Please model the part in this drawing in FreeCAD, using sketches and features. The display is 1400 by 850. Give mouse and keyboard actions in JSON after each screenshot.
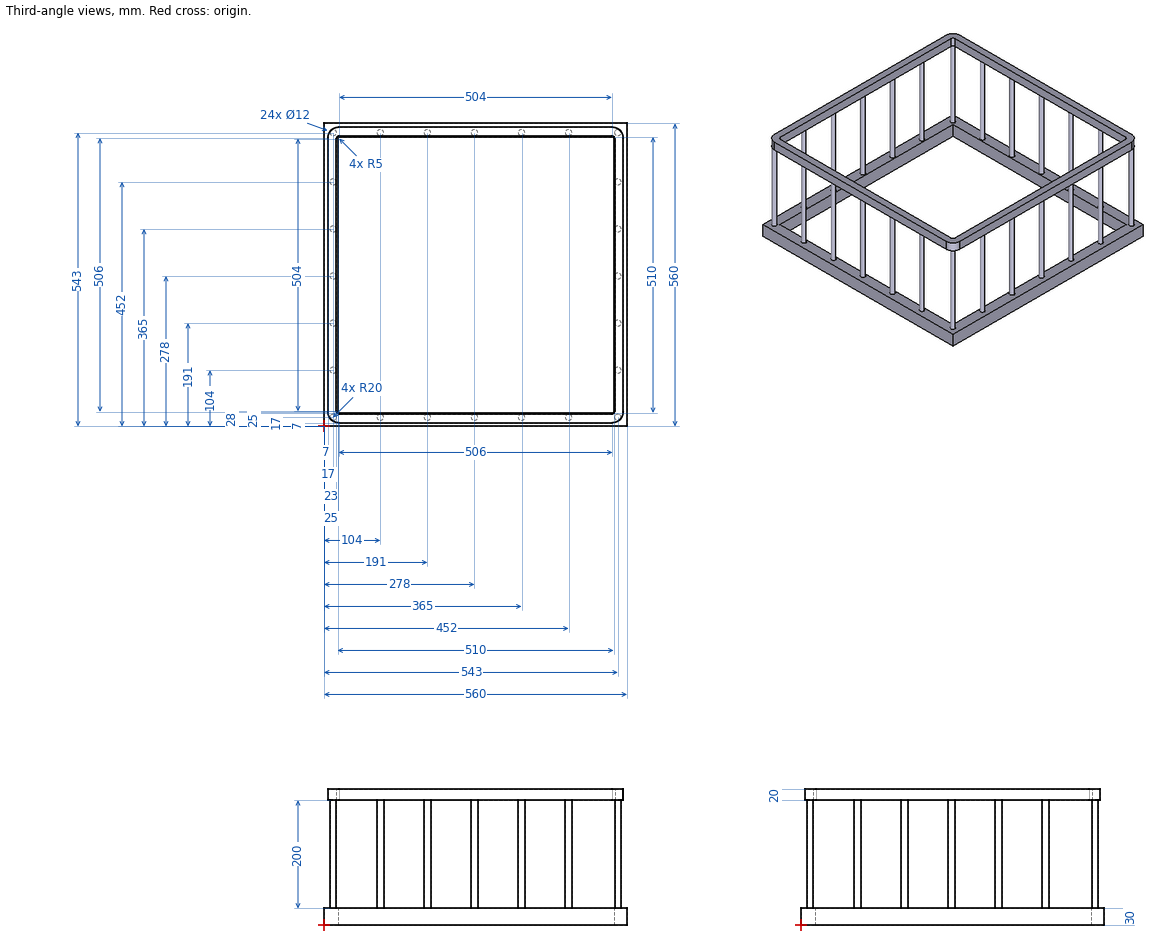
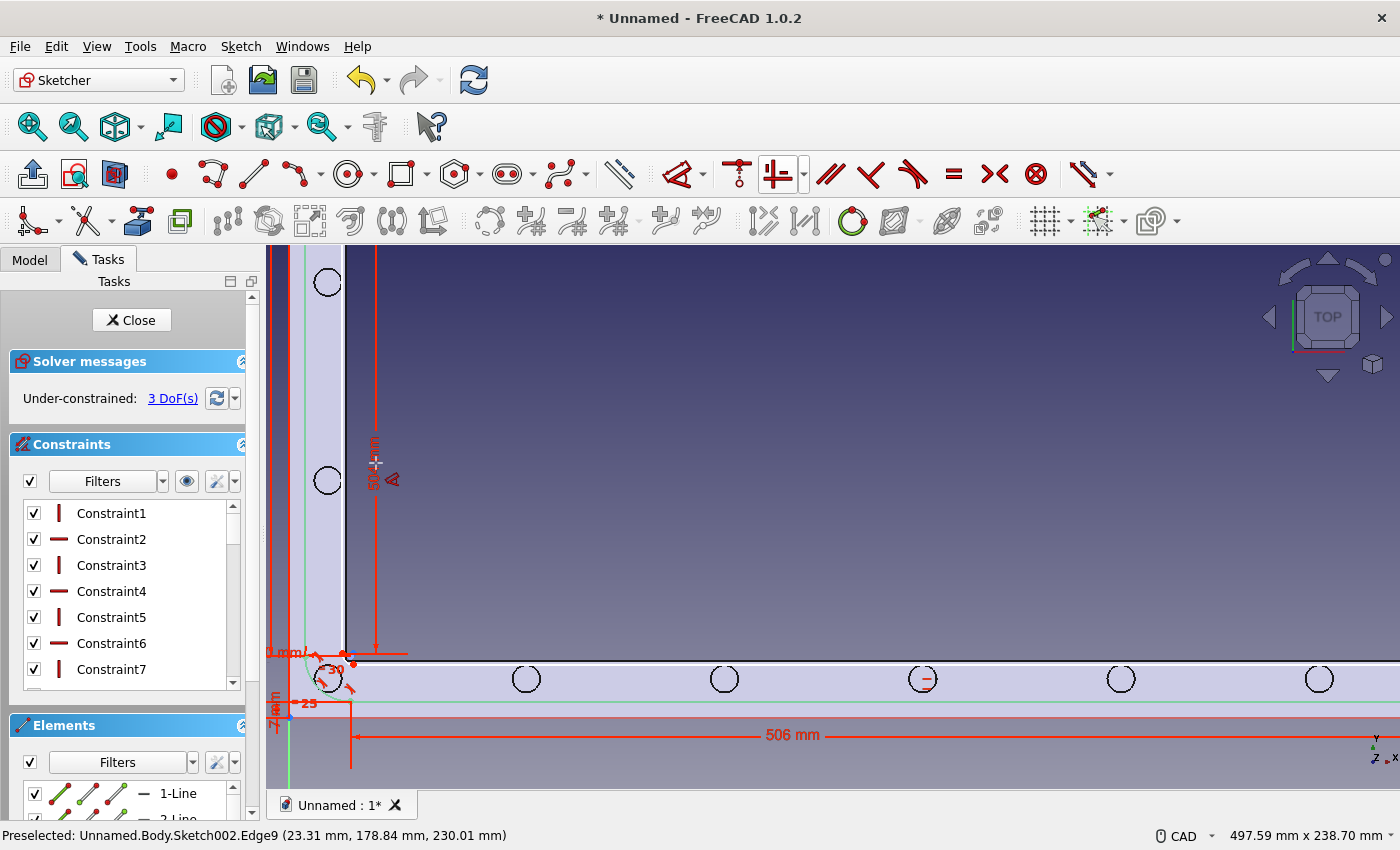
{"action": "scroll", "coordinate": [698, 702], "scroll_direction": "down", "scroll_amount": 6}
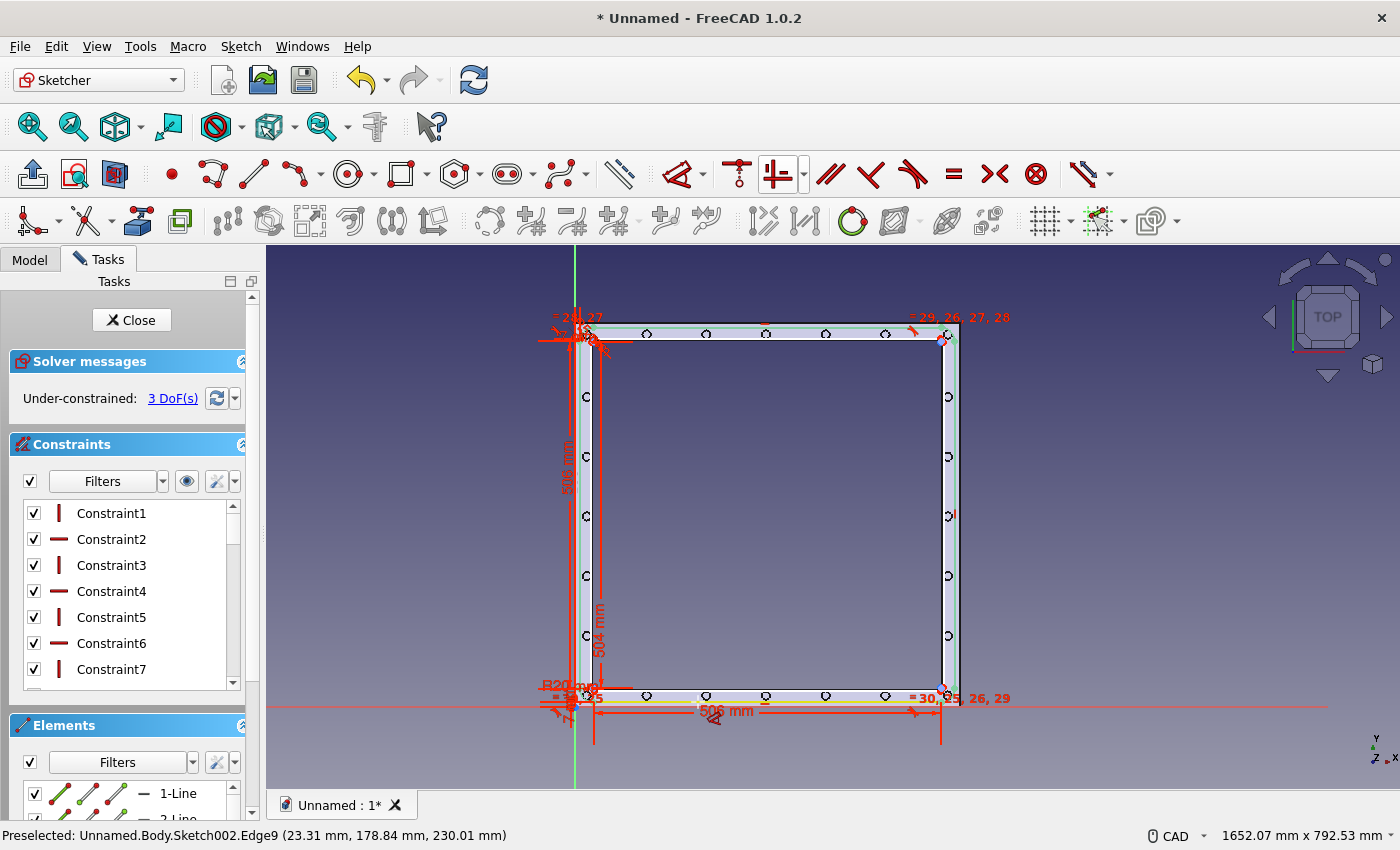
{"action": "scroll", "coordinate": [698, 339], "scroll_direction": "up", "scroll_amount": 2}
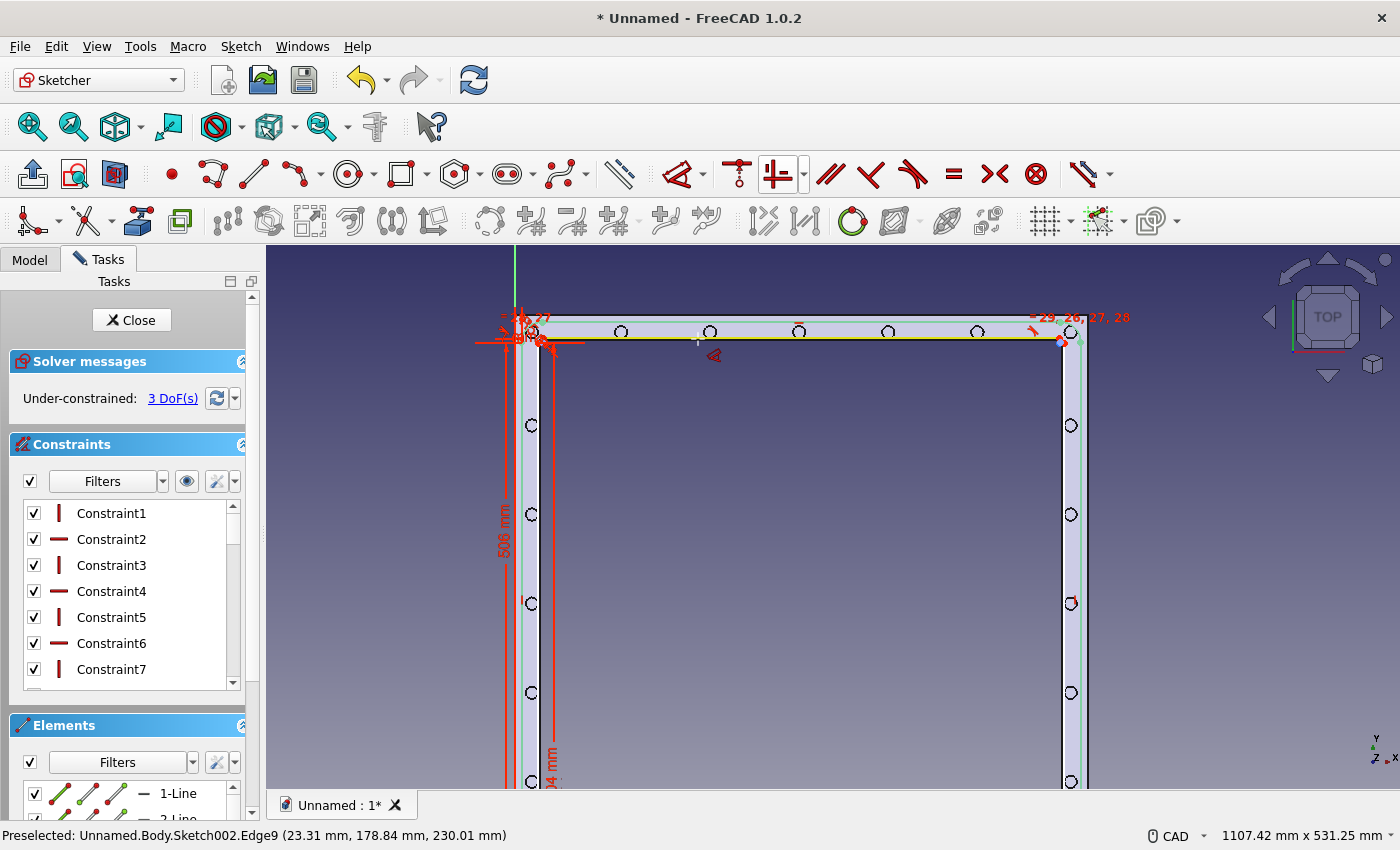
{"action": "left_click", "coordinate": [698, 338]}
{"action": "left_click", "coordinate": [801, 304]}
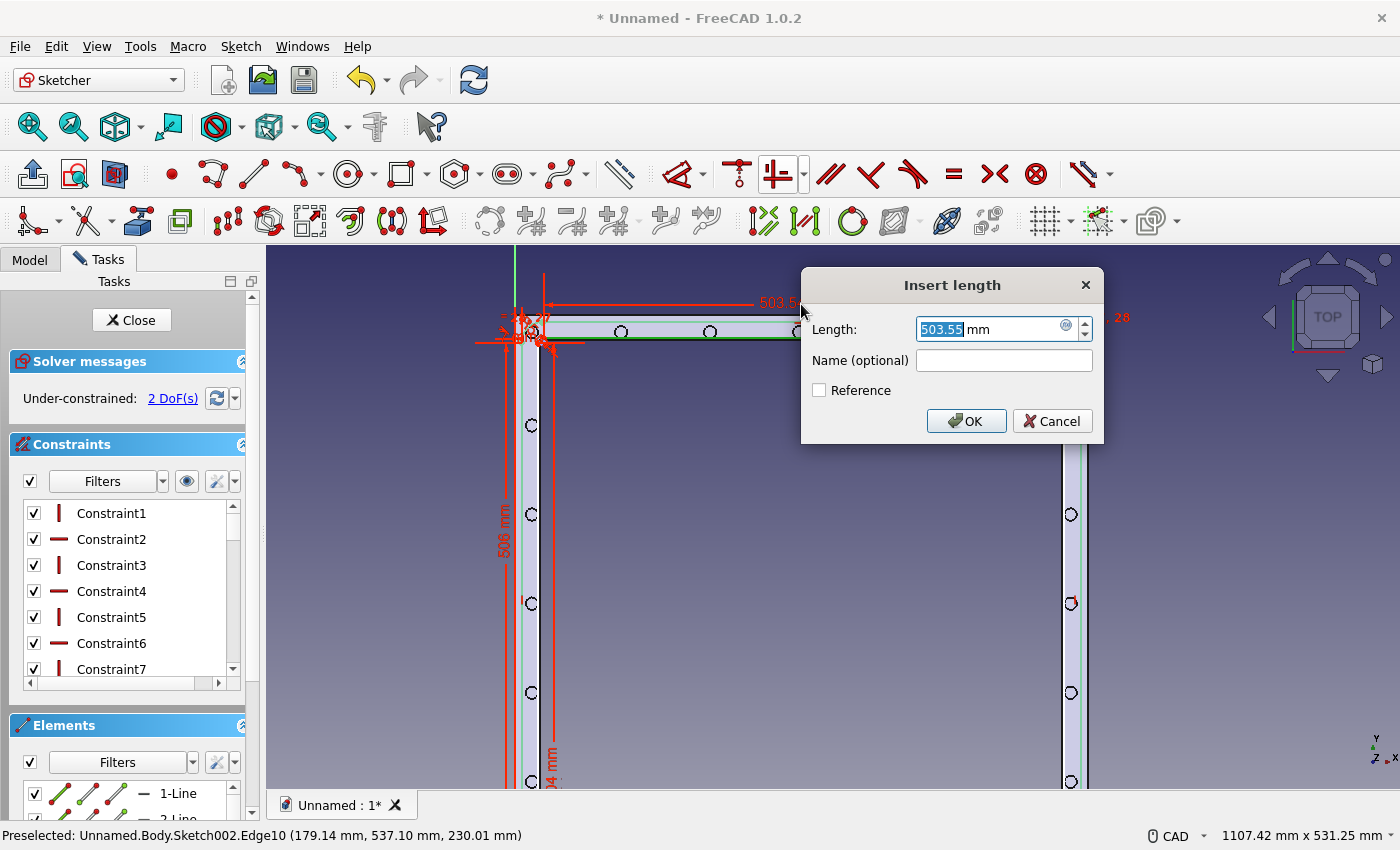
{"action": "type", "text": "504"}
{"action": "key", "text": "Return"}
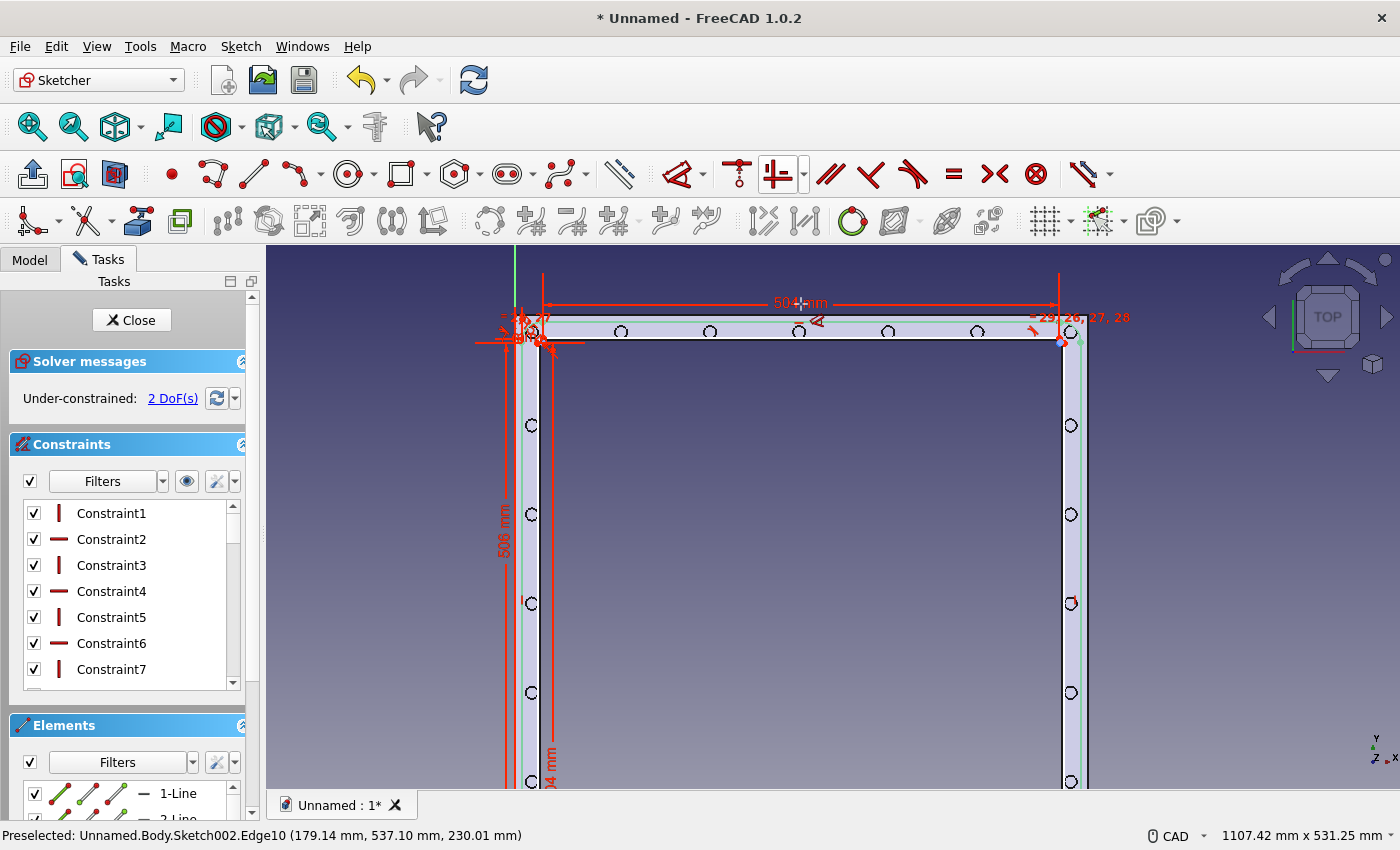
{"action": "scroll", "coordinate": [697, 338], "scroll_direction": "down", "scroll_amount": 2}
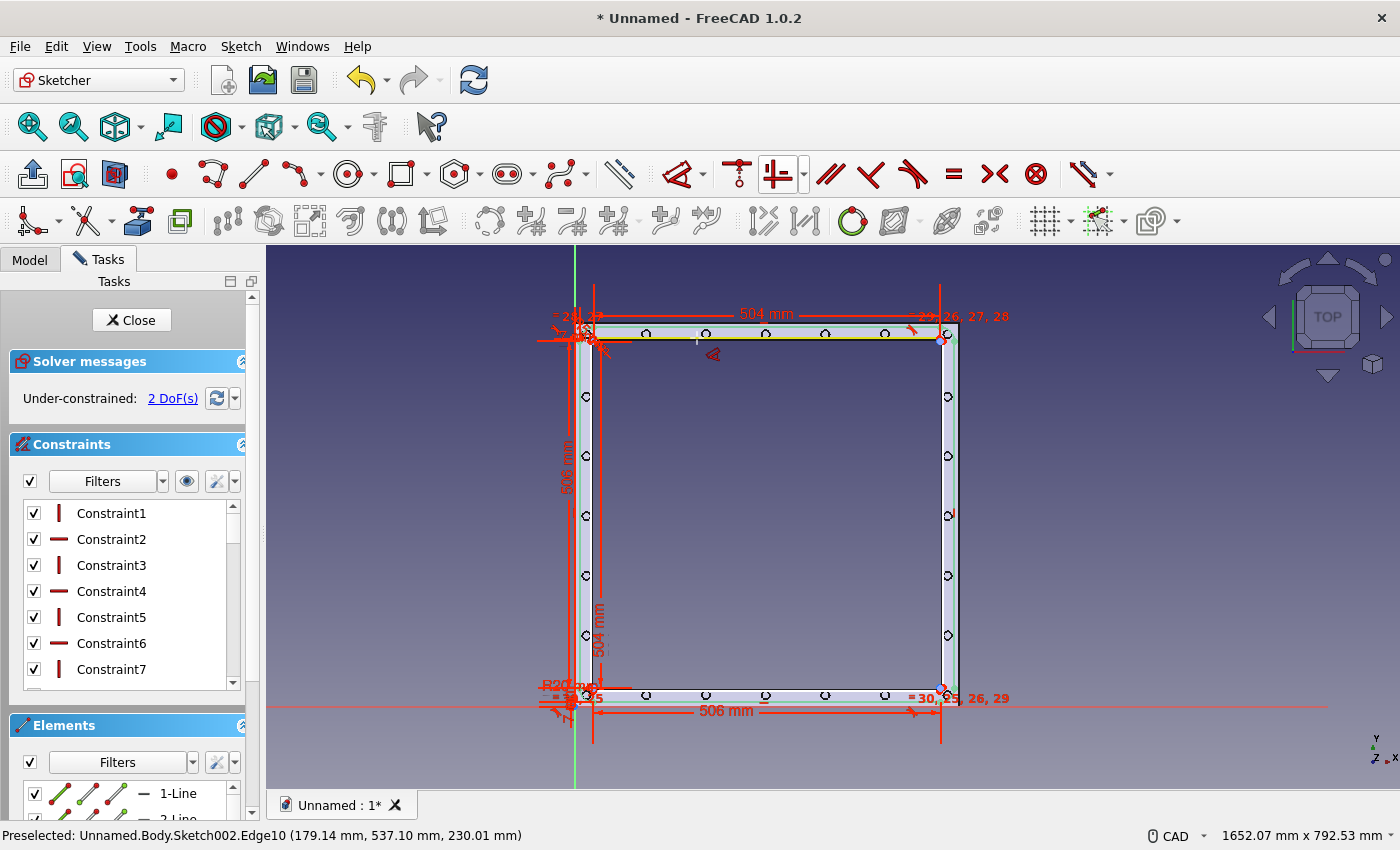
{"action": "scroll", "coordinate": [591, 688], "scroll_direction": "up", "scroll_amount": 8}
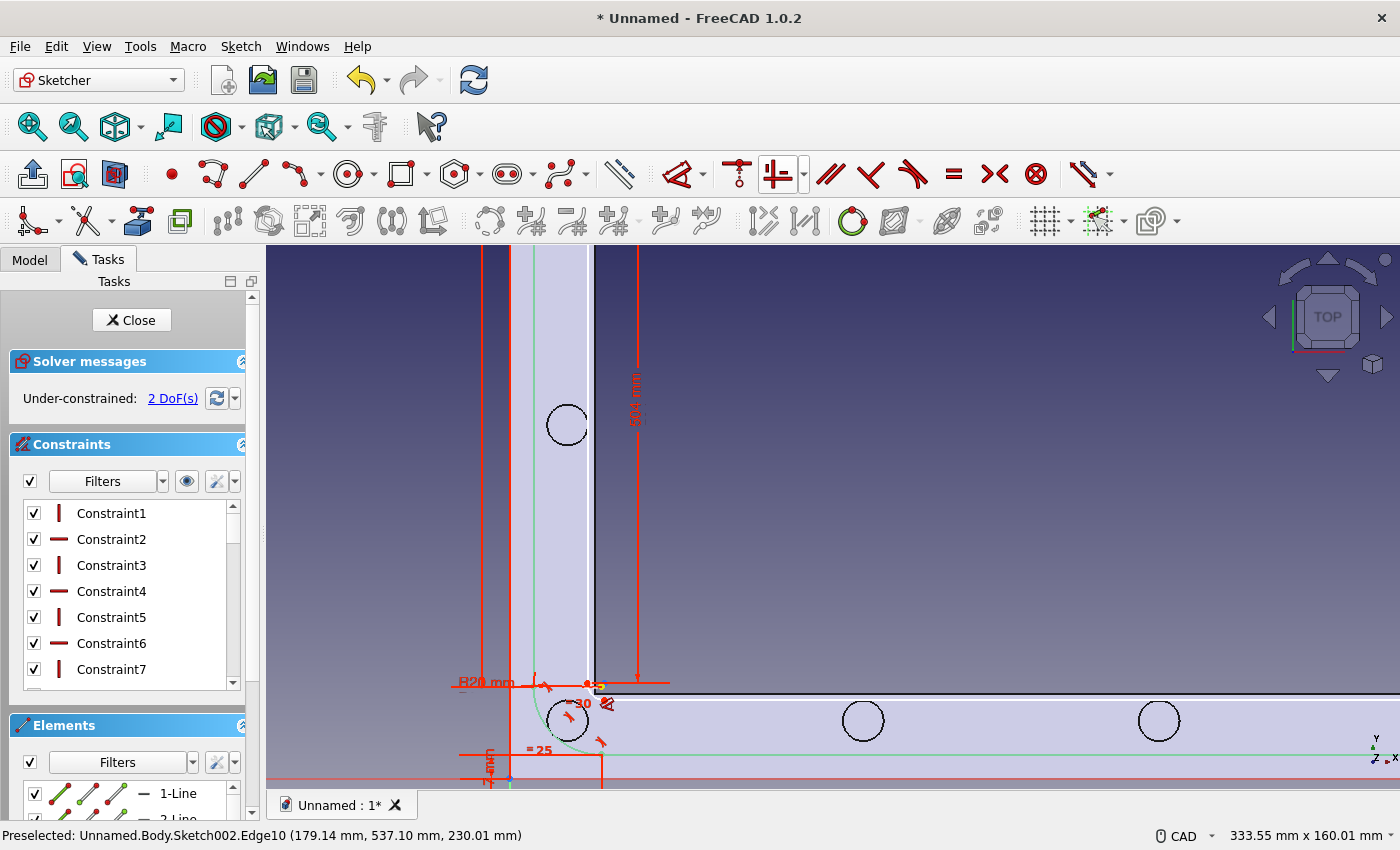
{"action": "left_click", "coordinate": [588, 683]}
{"action": "left_click", "coordinate": [549, 649]}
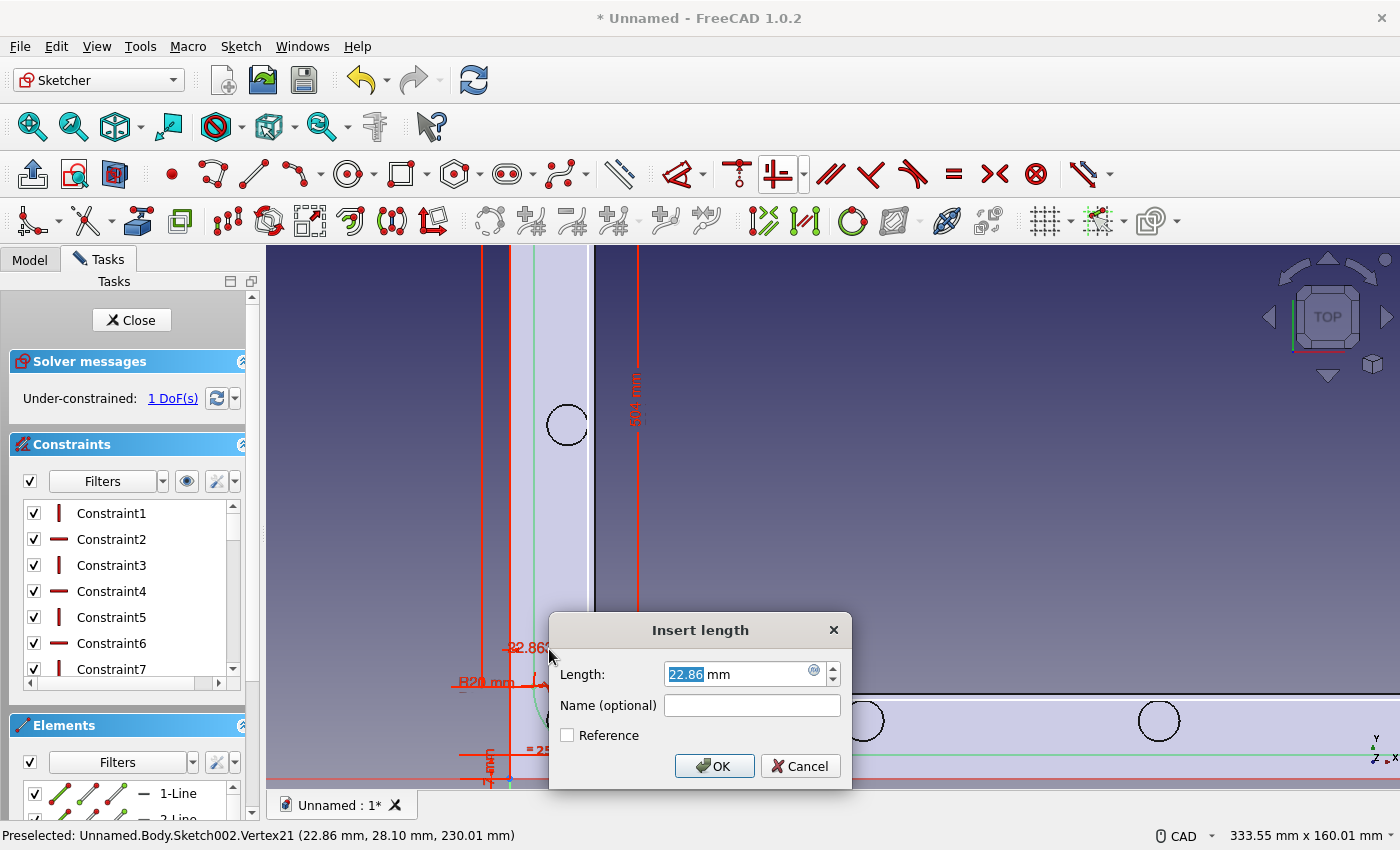
{"action": "type", "text": "23"}
{"action": "key", "text": "Return"}